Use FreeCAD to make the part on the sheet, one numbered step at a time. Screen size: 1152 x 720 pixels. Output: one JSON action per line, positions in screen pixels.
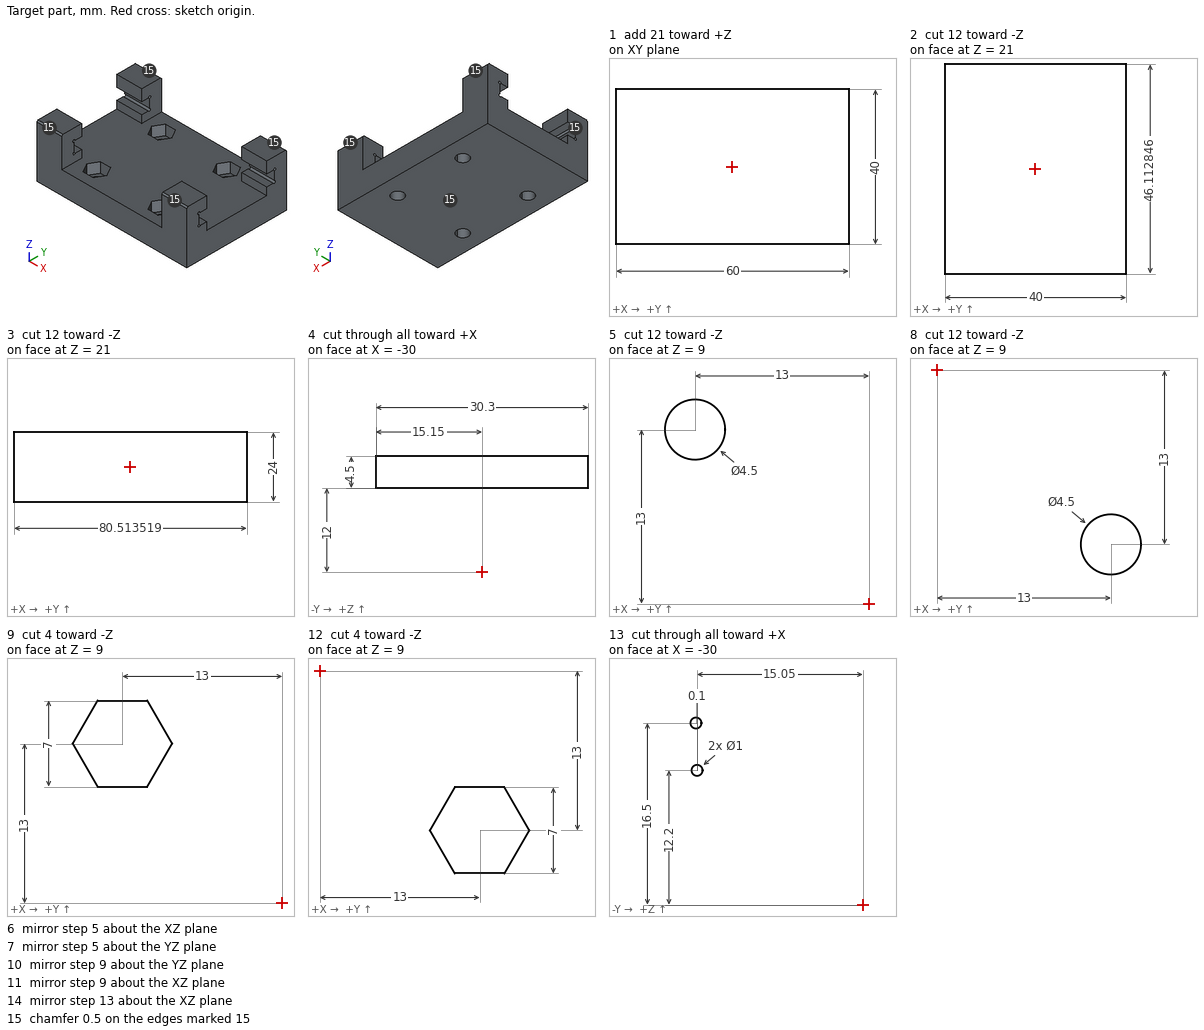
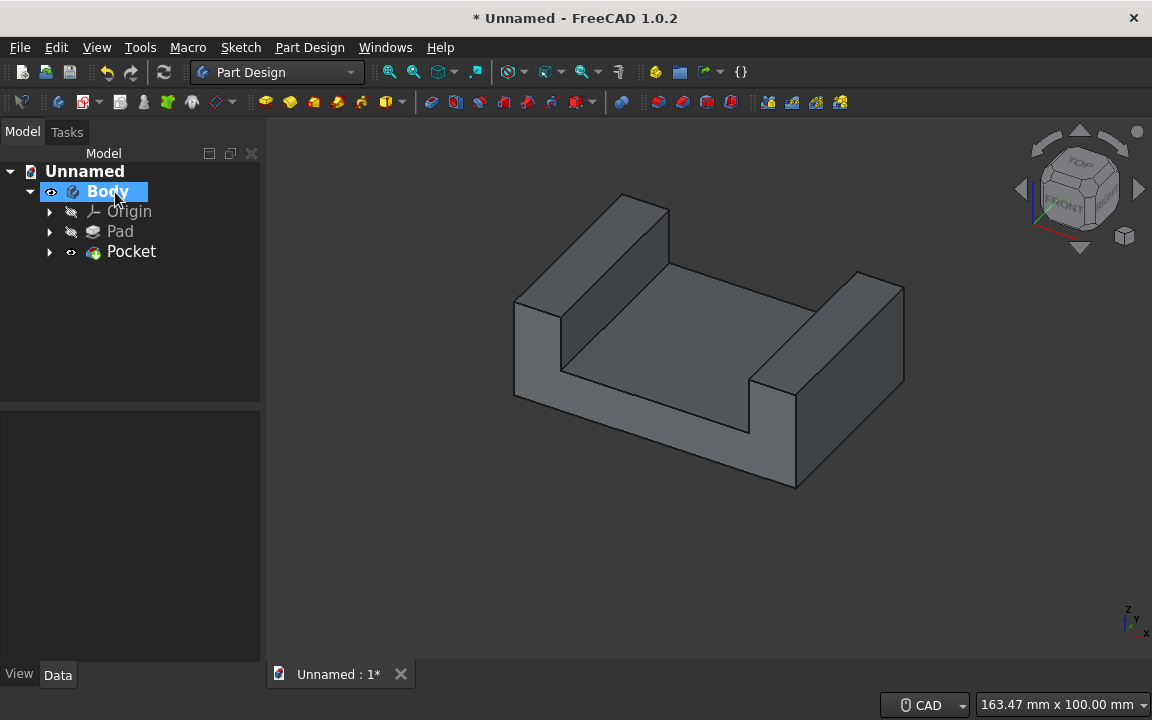
{"action": "left_click", "coordinate": [623, 224]}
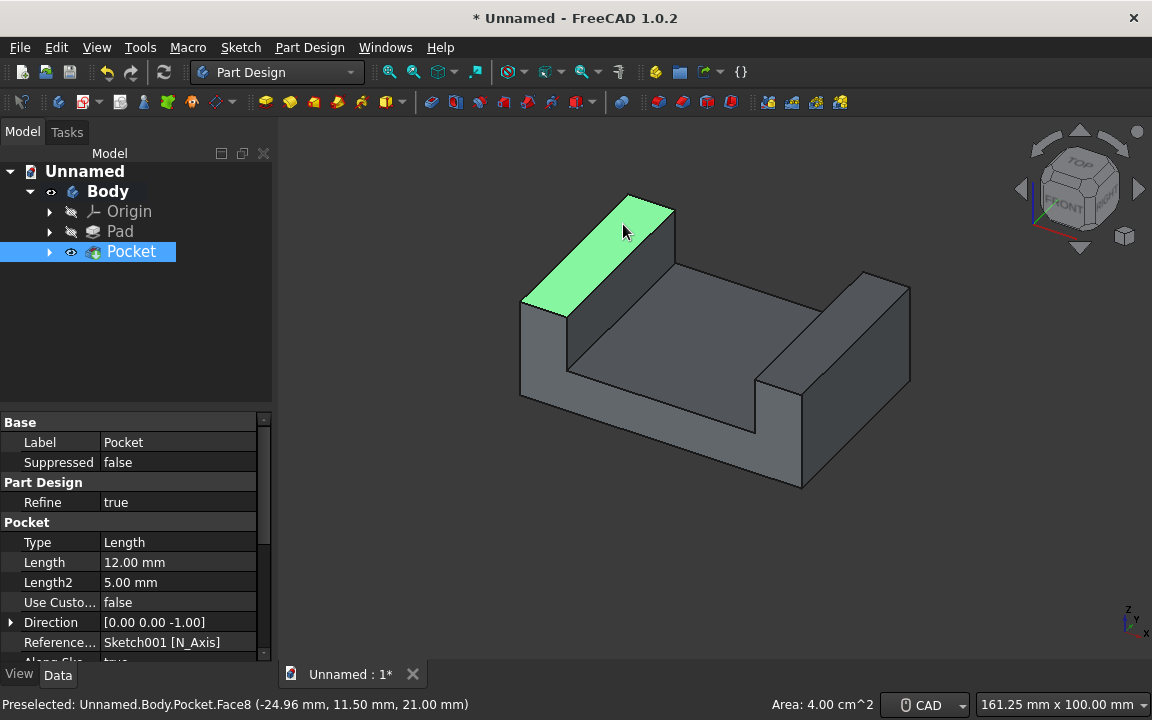
{"action": "left_click", "coordinate": [84, 102]}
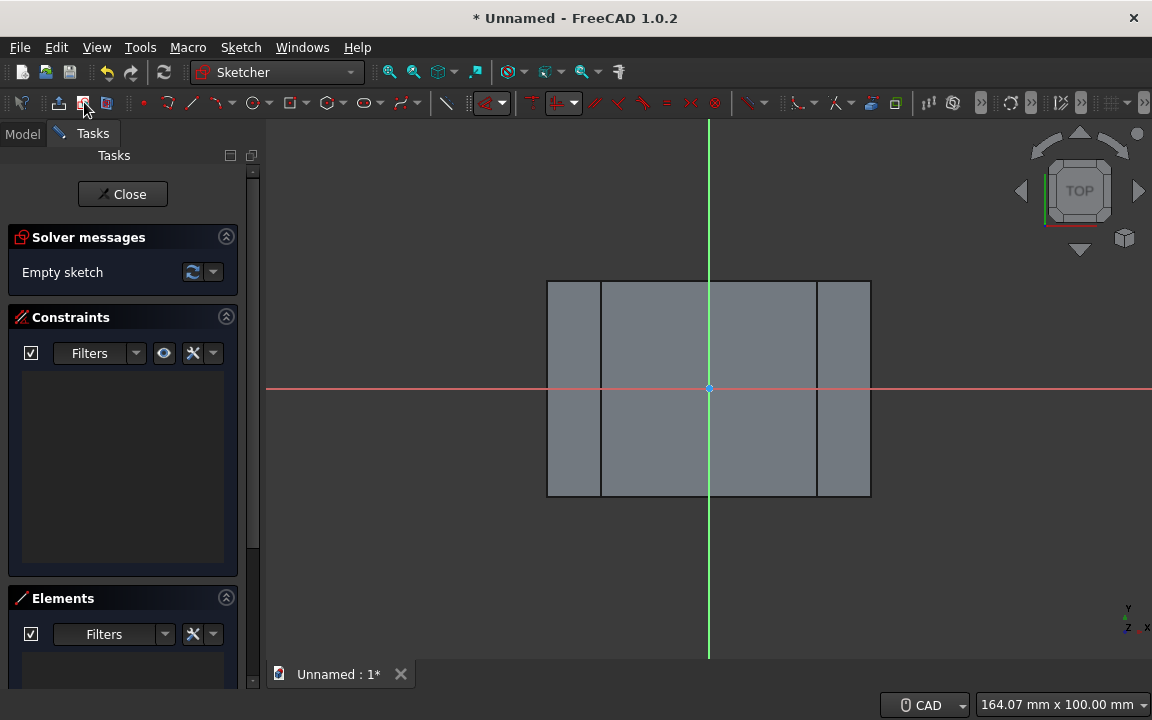
{"action": "left_click", "coordinate": [290, 104]}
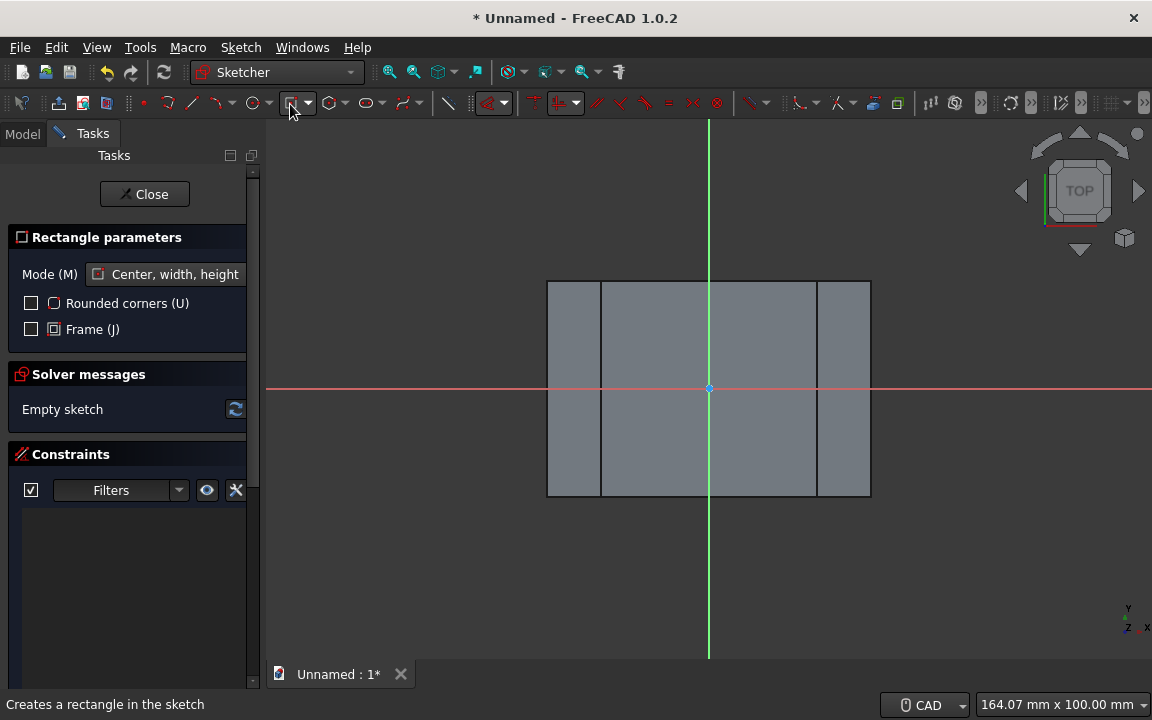
{"action": "left_click", "coordinate": [709, 389]}
{"action": "left_click", "coordinate": [926, 324]}
{"action": "key", "text": "Escape"}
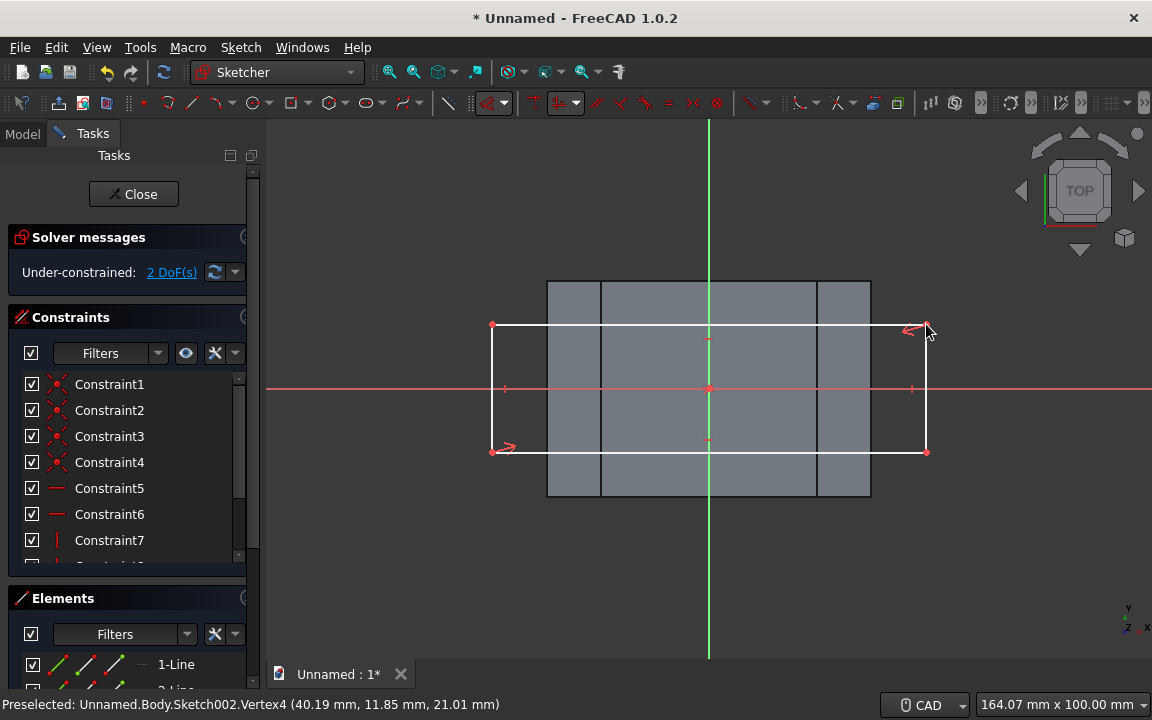
{"action": "left_click", "coordinate": [926, 415]}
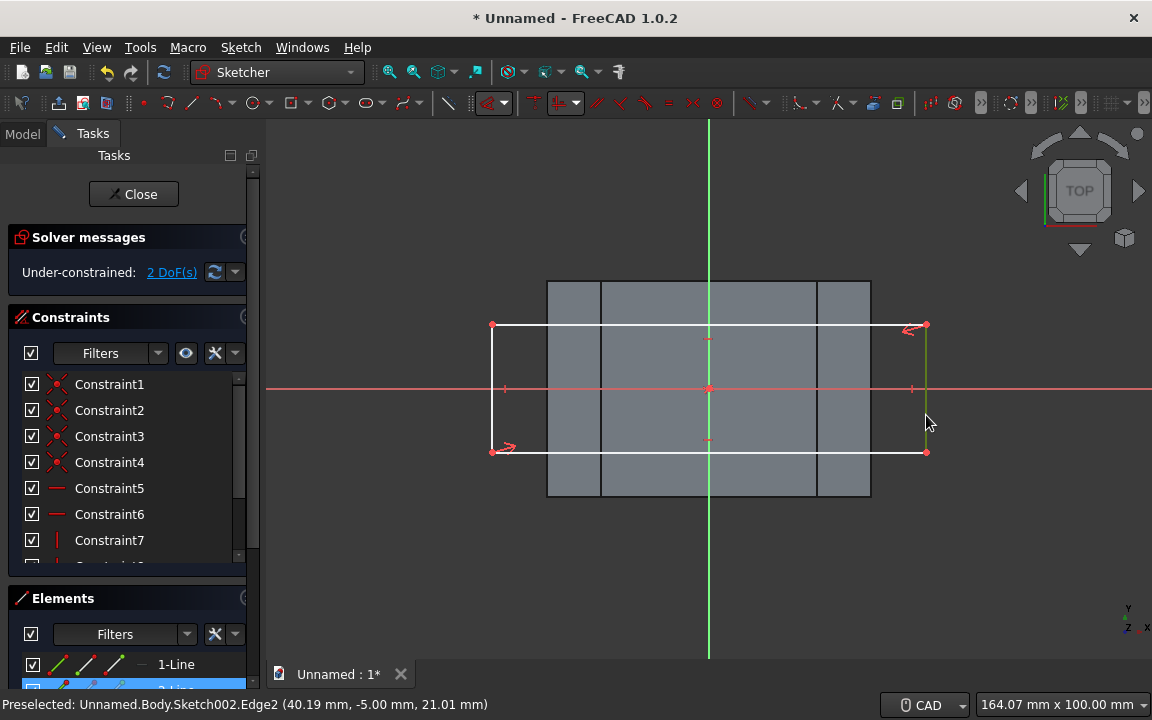
{"action": "key", "text": "i"}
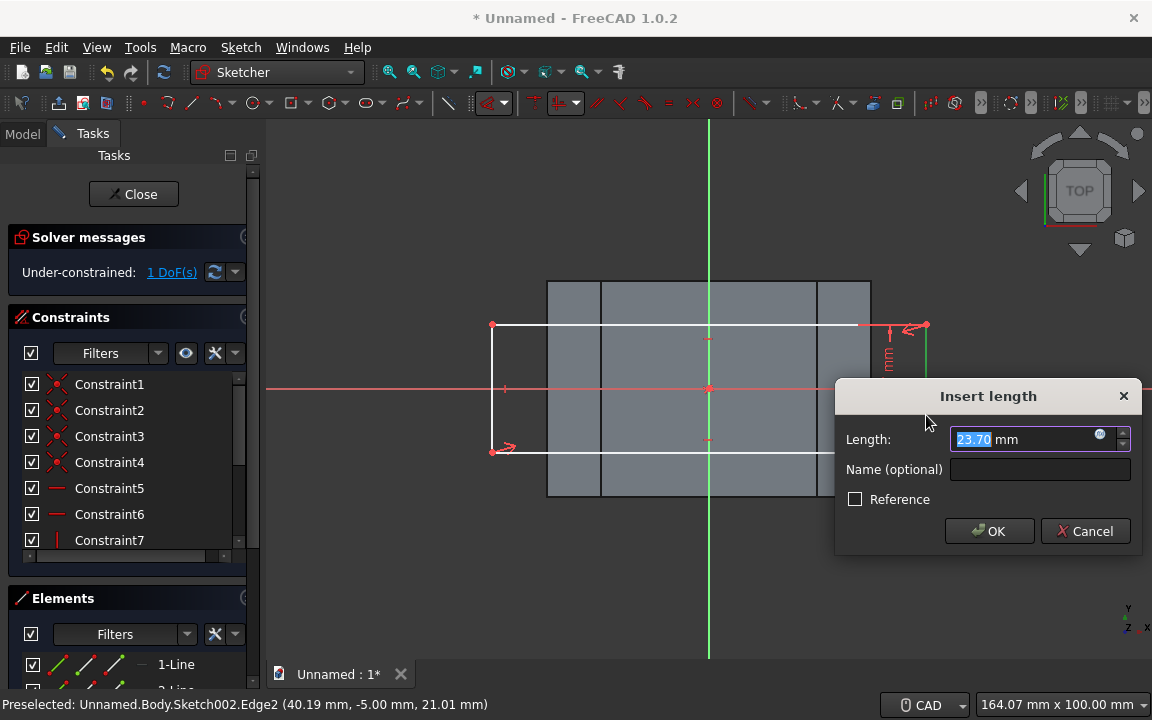
{"action": "type", "text": "24"}
{"action": "key", "text": "Return"}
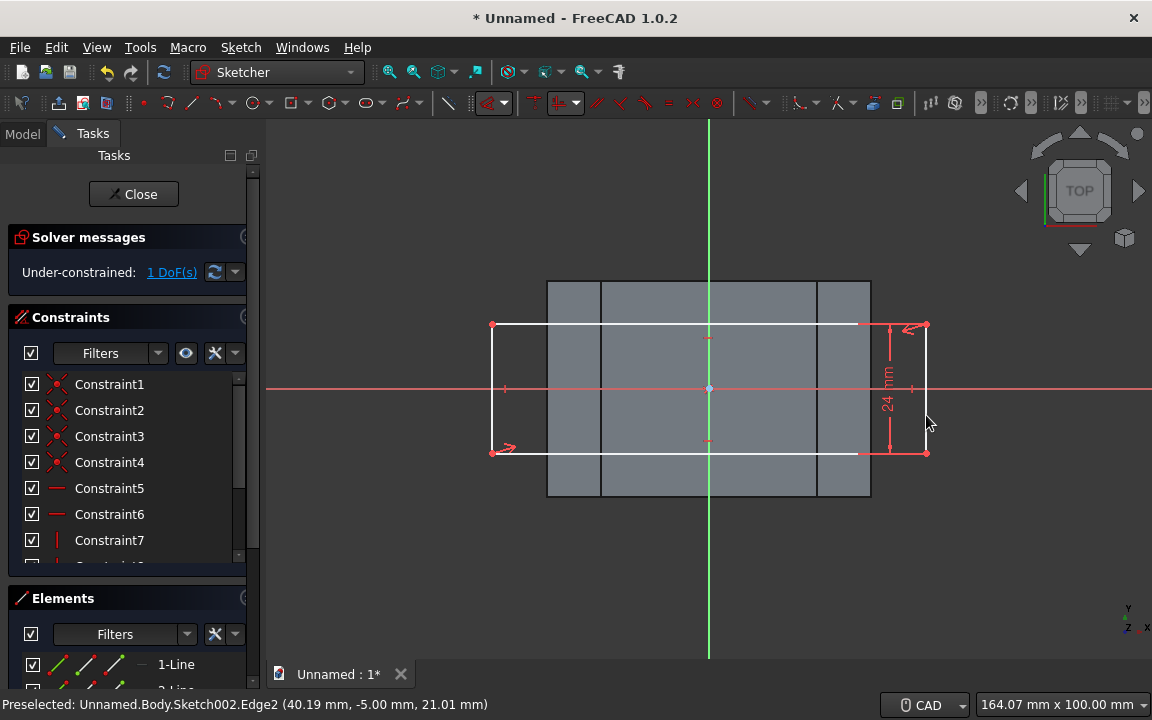
{"action": "left_click", "coordinate": [622, 454]}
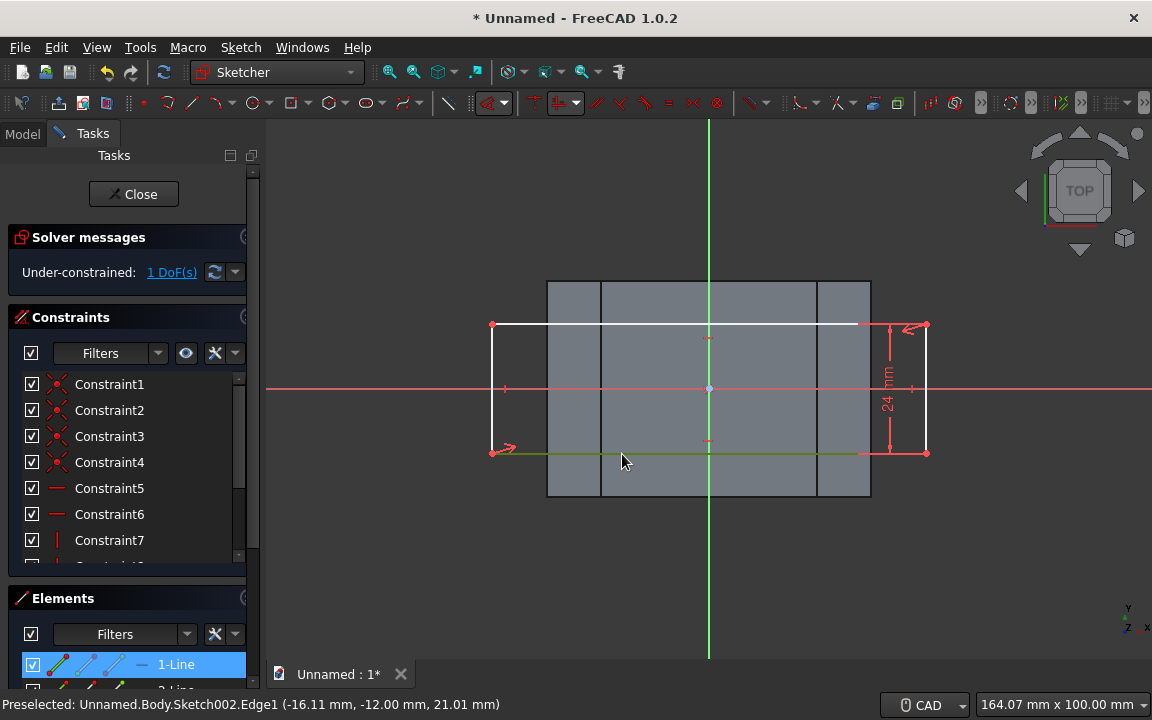
{"action": "key", "text": "l"}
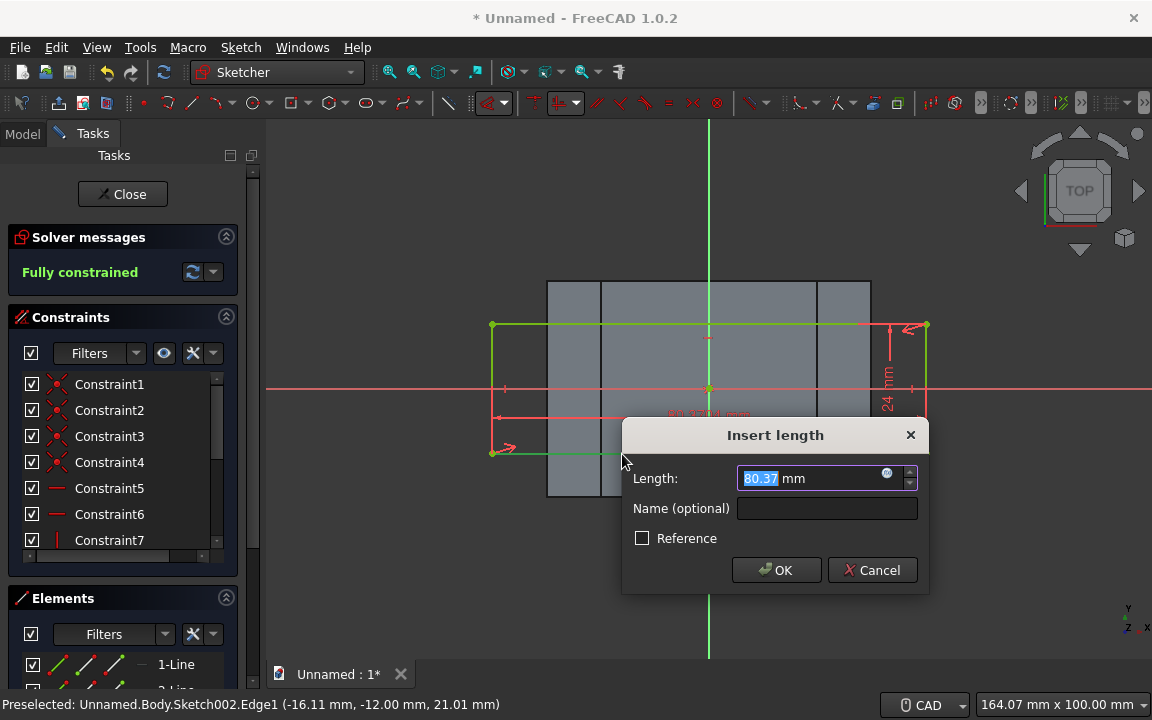
{"action": "type", "text": "80.513519"}
{"action": "key", "text": "Return"}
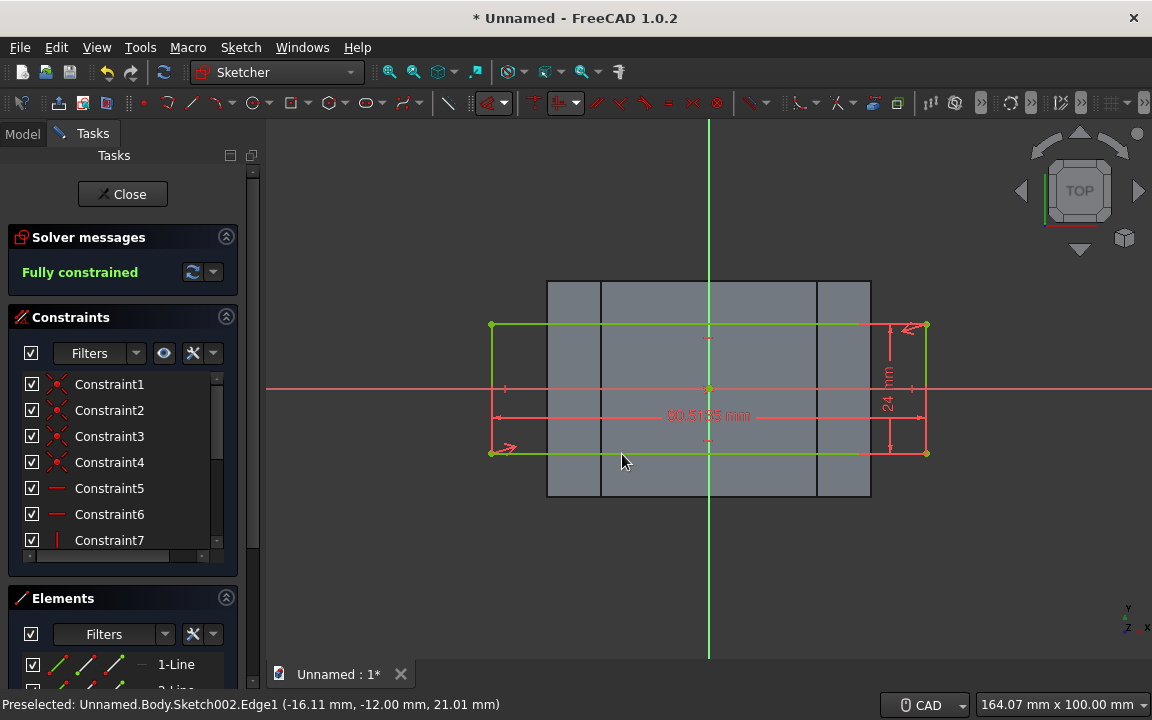
{"action": "left_click", "coordinate": [123, 194]}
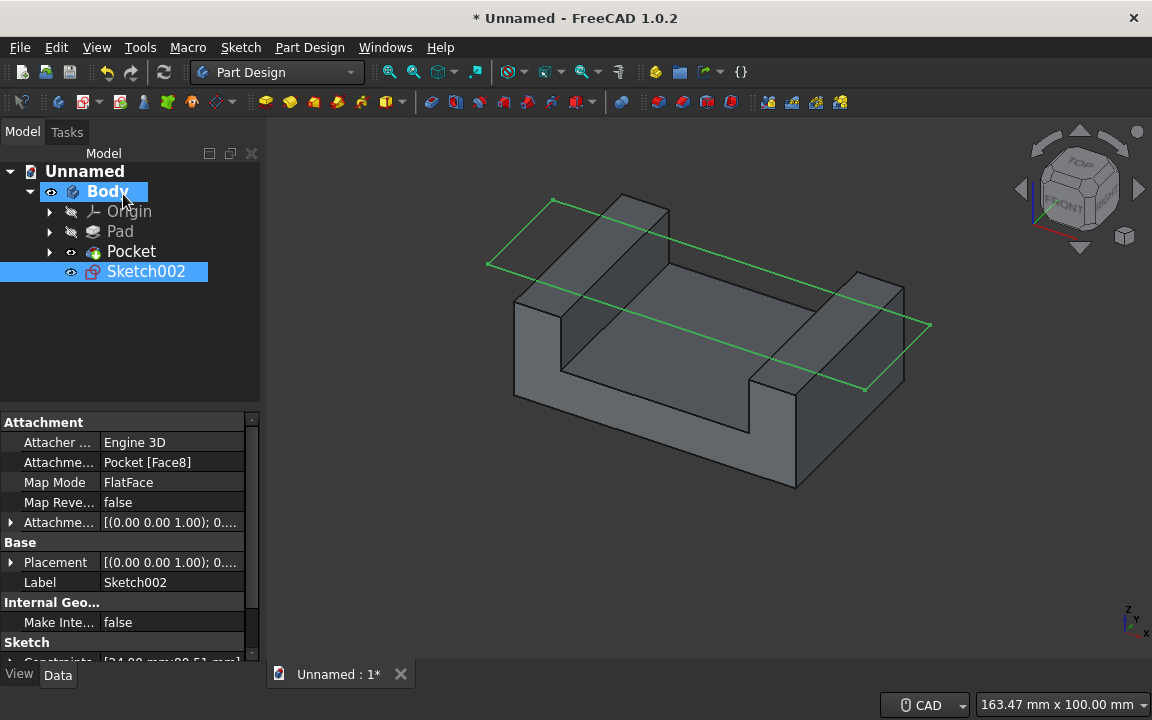
{"action": "left_click", "coordinate": [432, 102]}